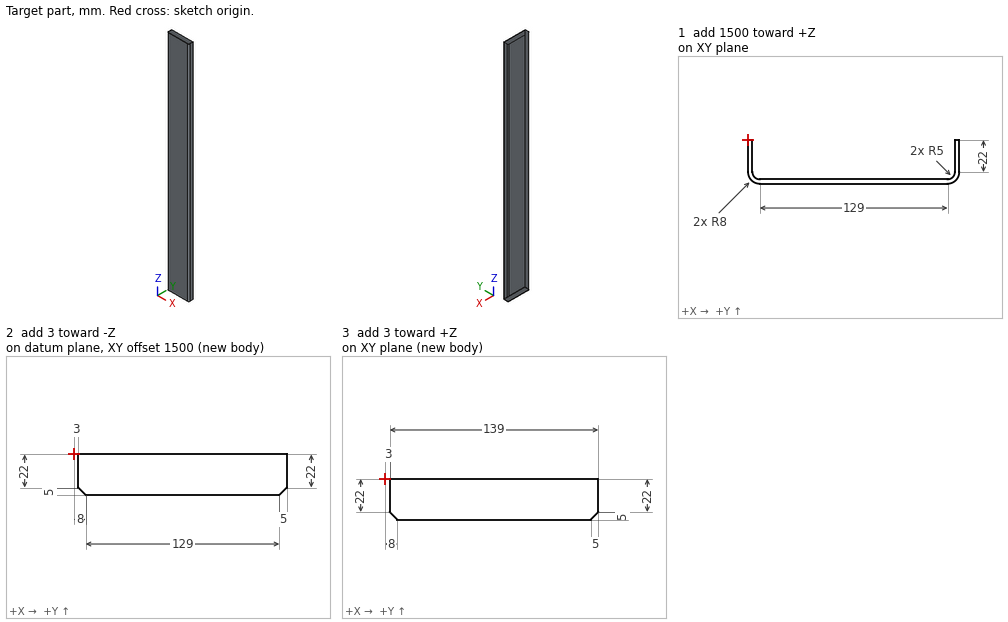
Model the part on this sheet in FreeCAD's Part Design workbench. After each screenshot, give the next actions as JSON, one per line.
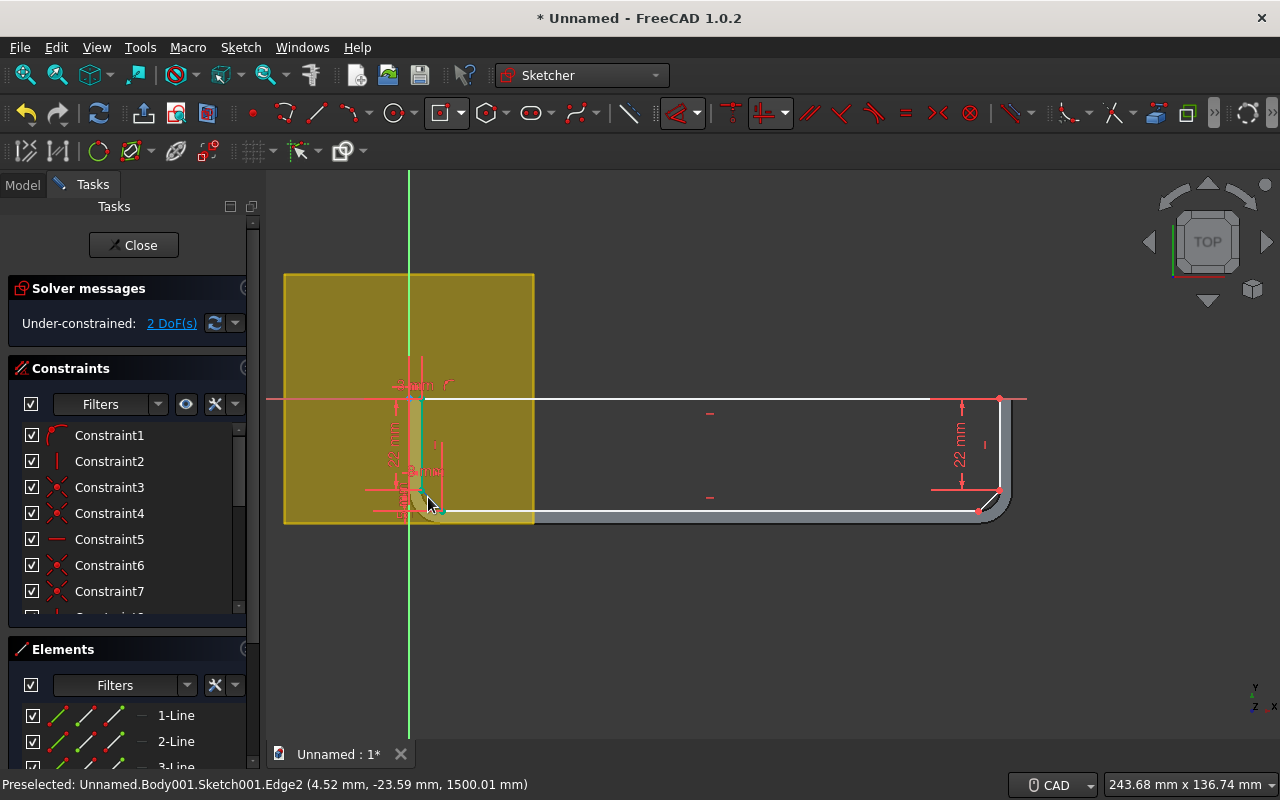
{"action": "scroll", "coordinate": [985, 505], "scroll_direction": "up", "scroll_amount": 4}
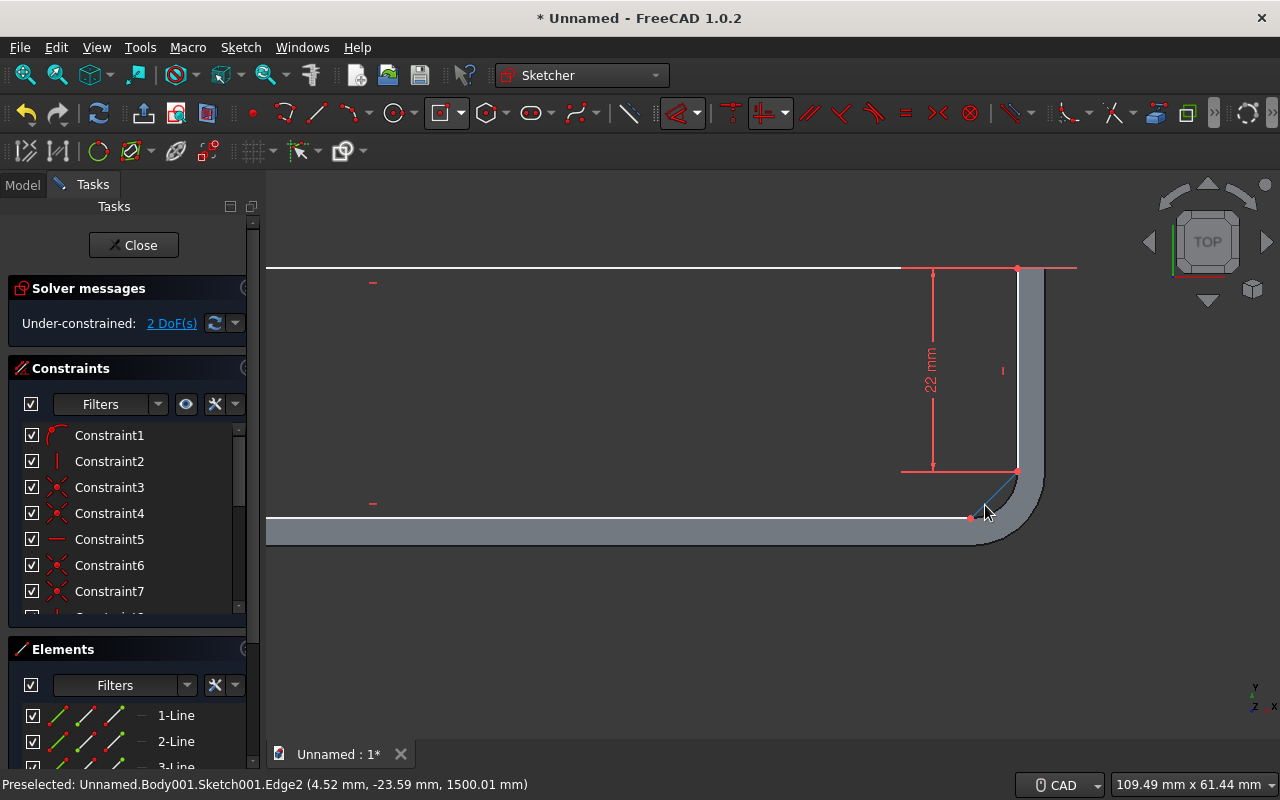
{"action": "left_click", "coordinate": [985, 504]}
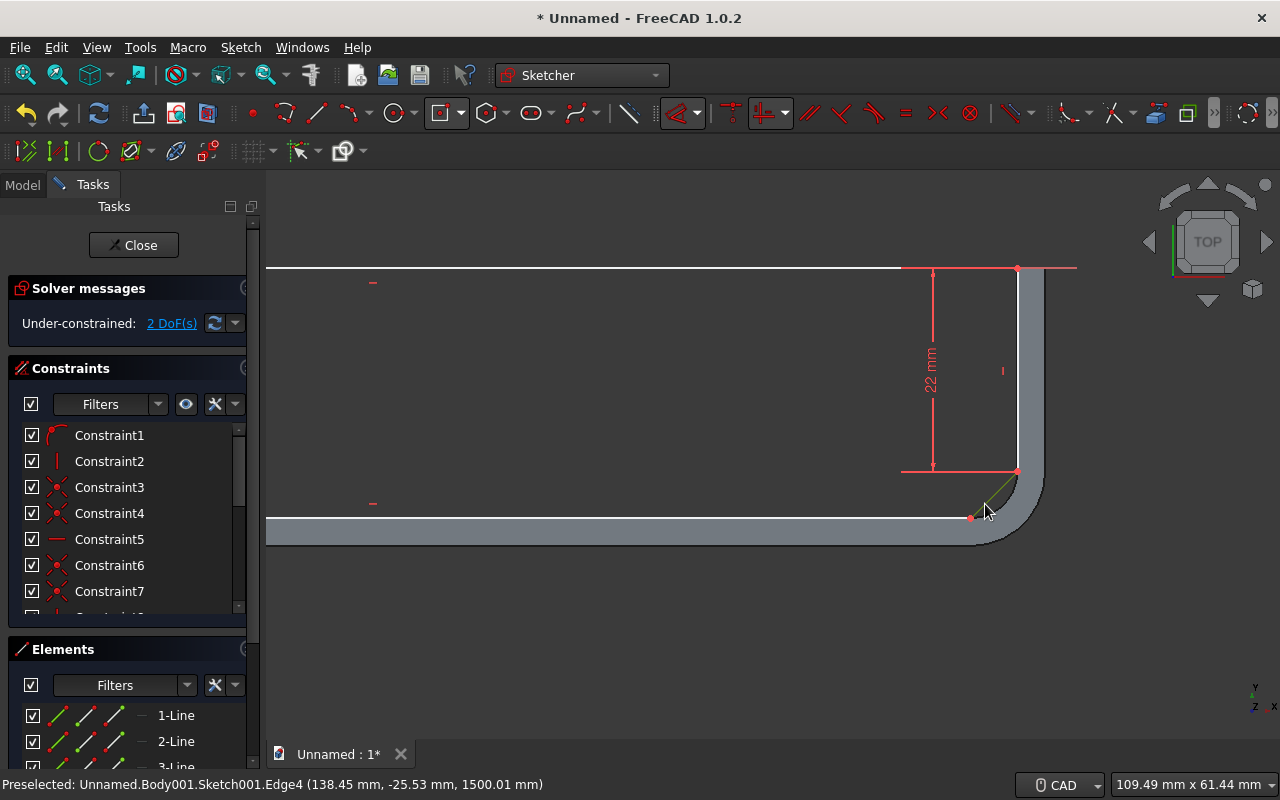
{"action": "key", "text": "l"}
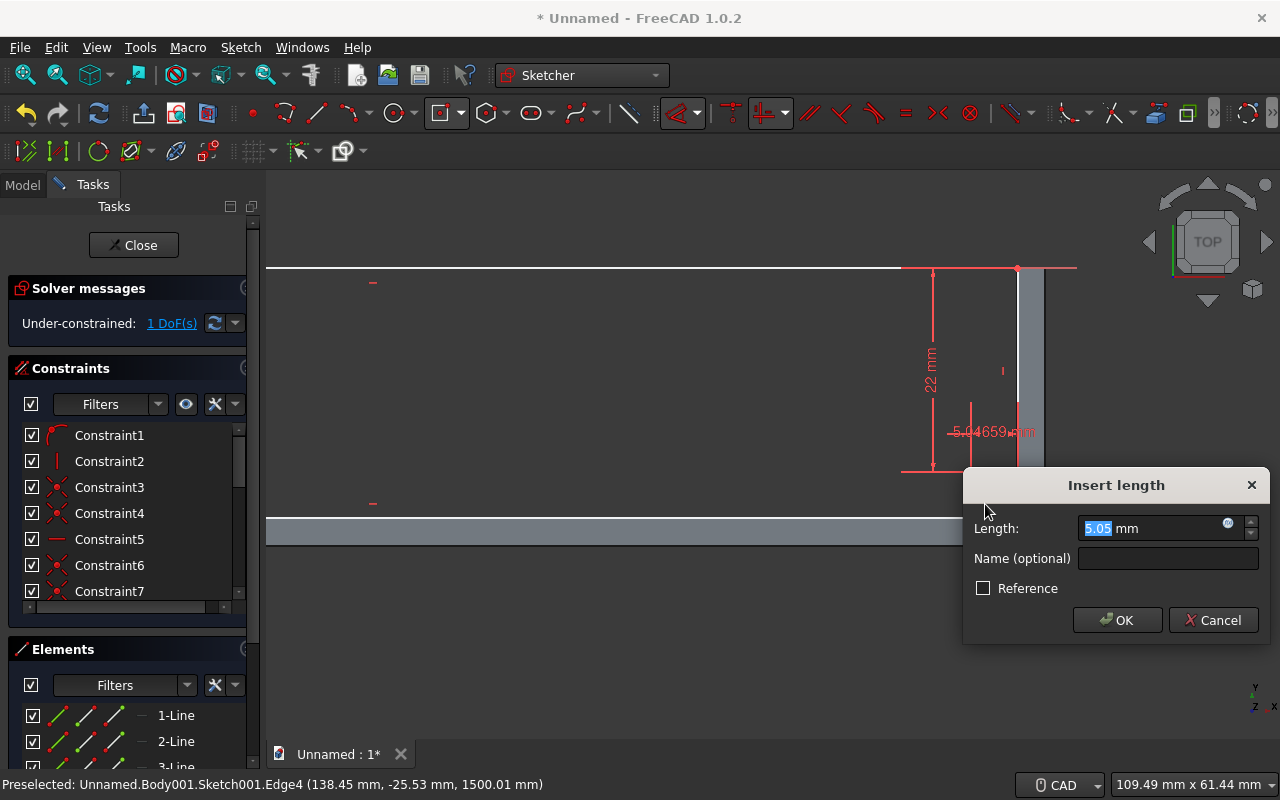
{"action": "type", "text": "5"}
{"action": "key", "text": "Return"}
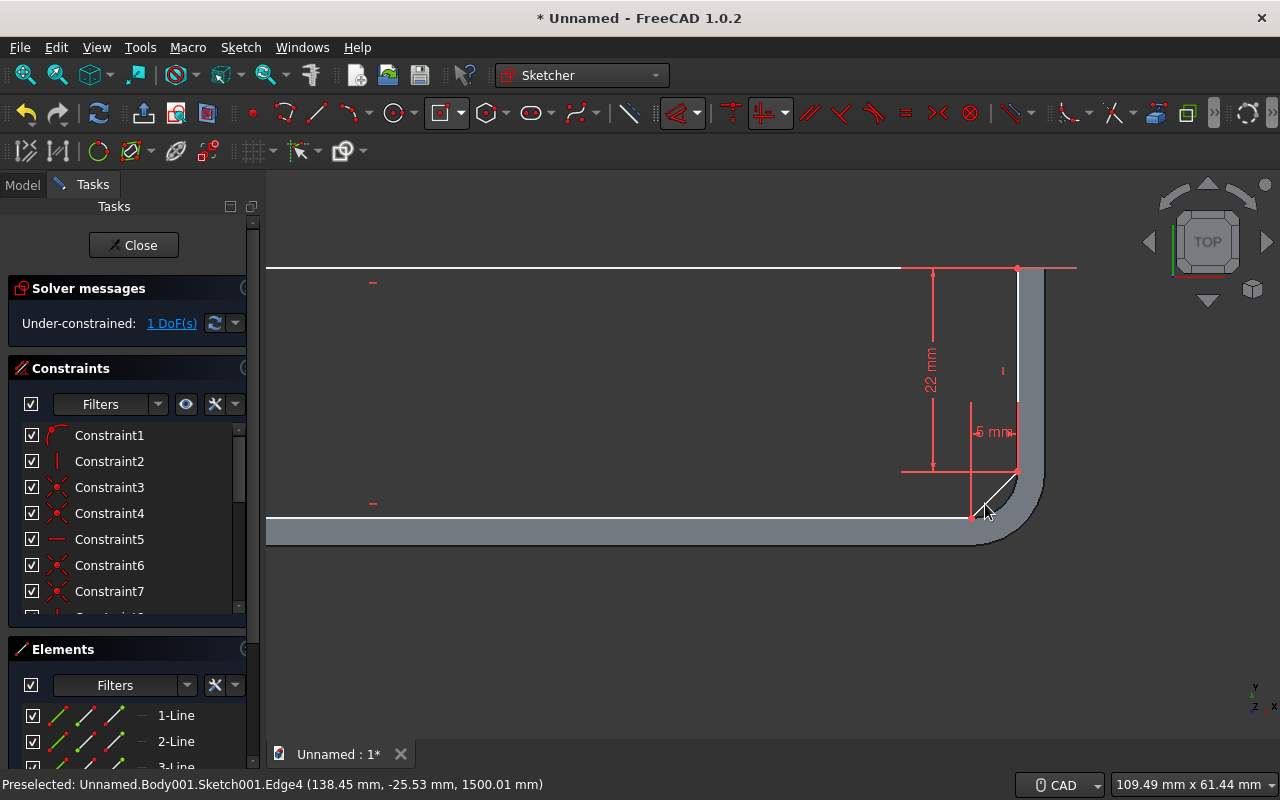
{"action": "left_click", "coordinate": [613, 518]}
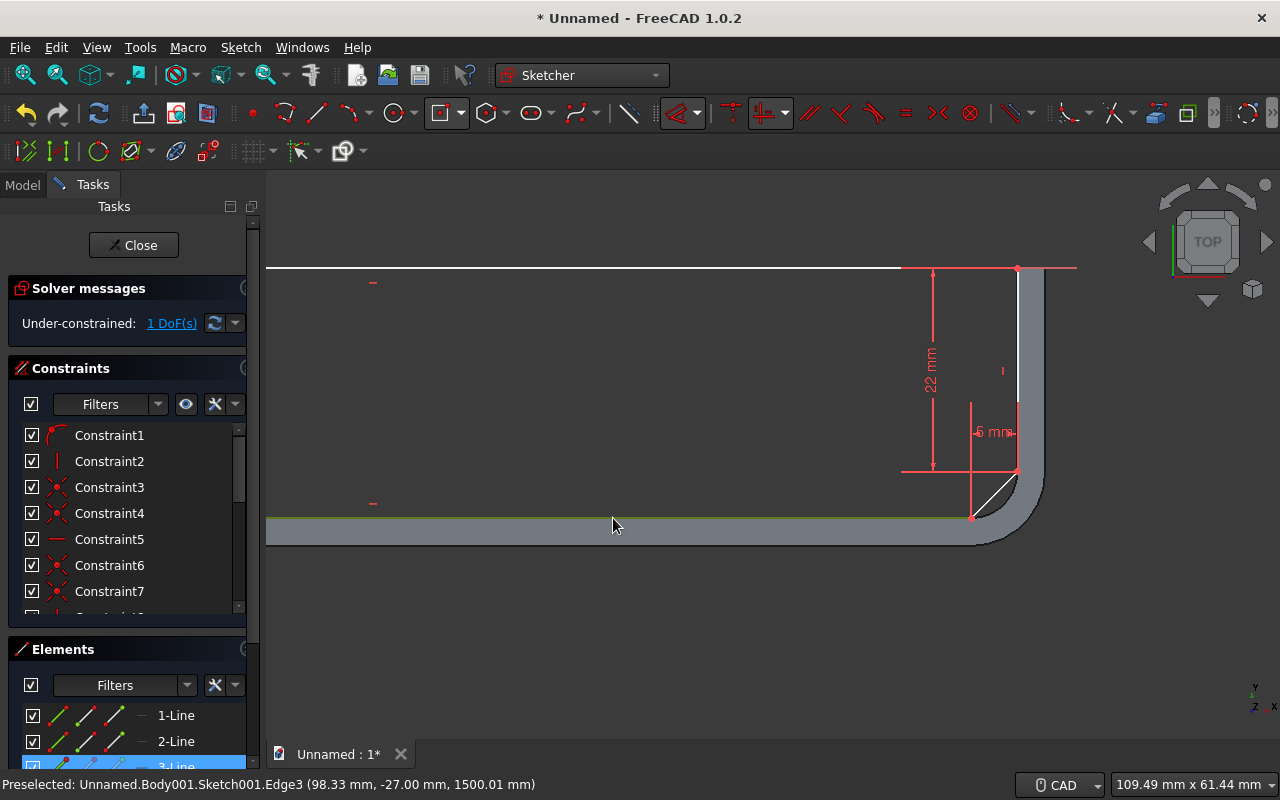
{"action": "key", "text": "l"}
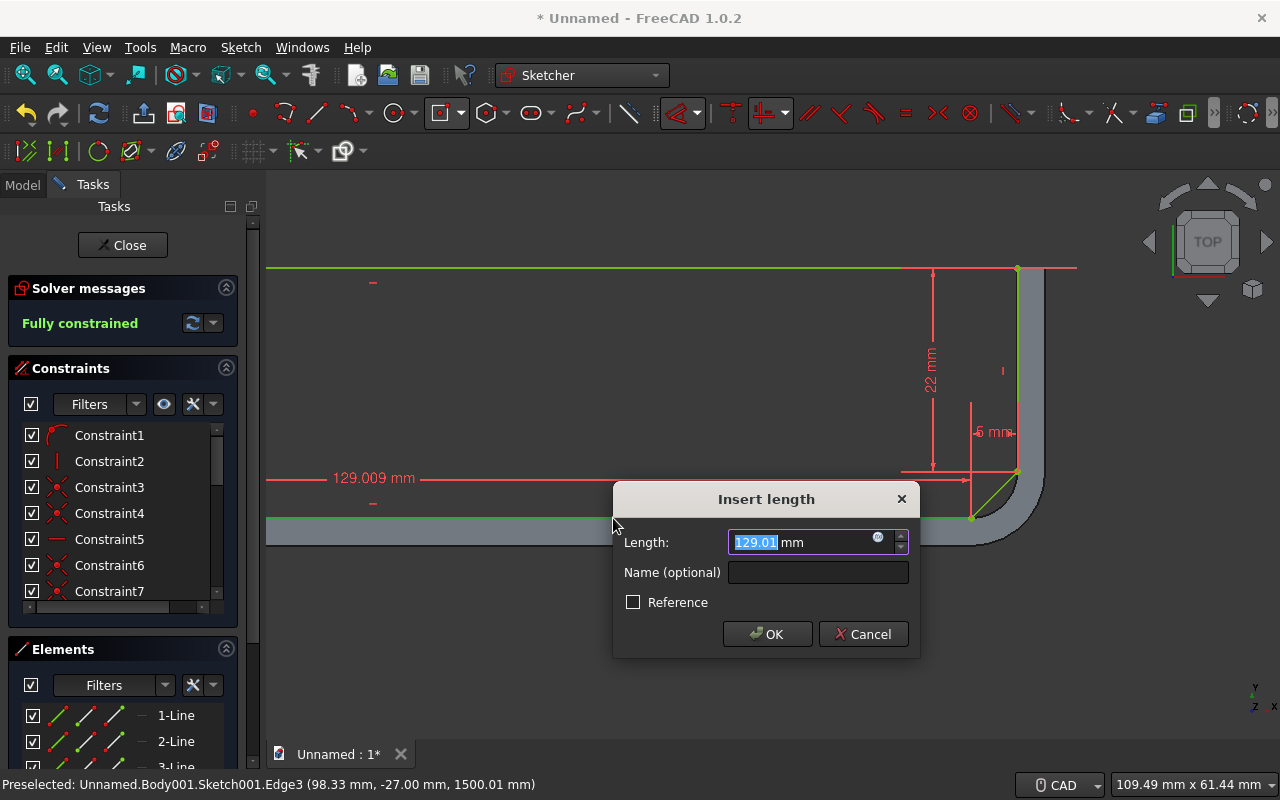
{"action": "type", "text": "129"}
{"action": "key", "text": "Return"}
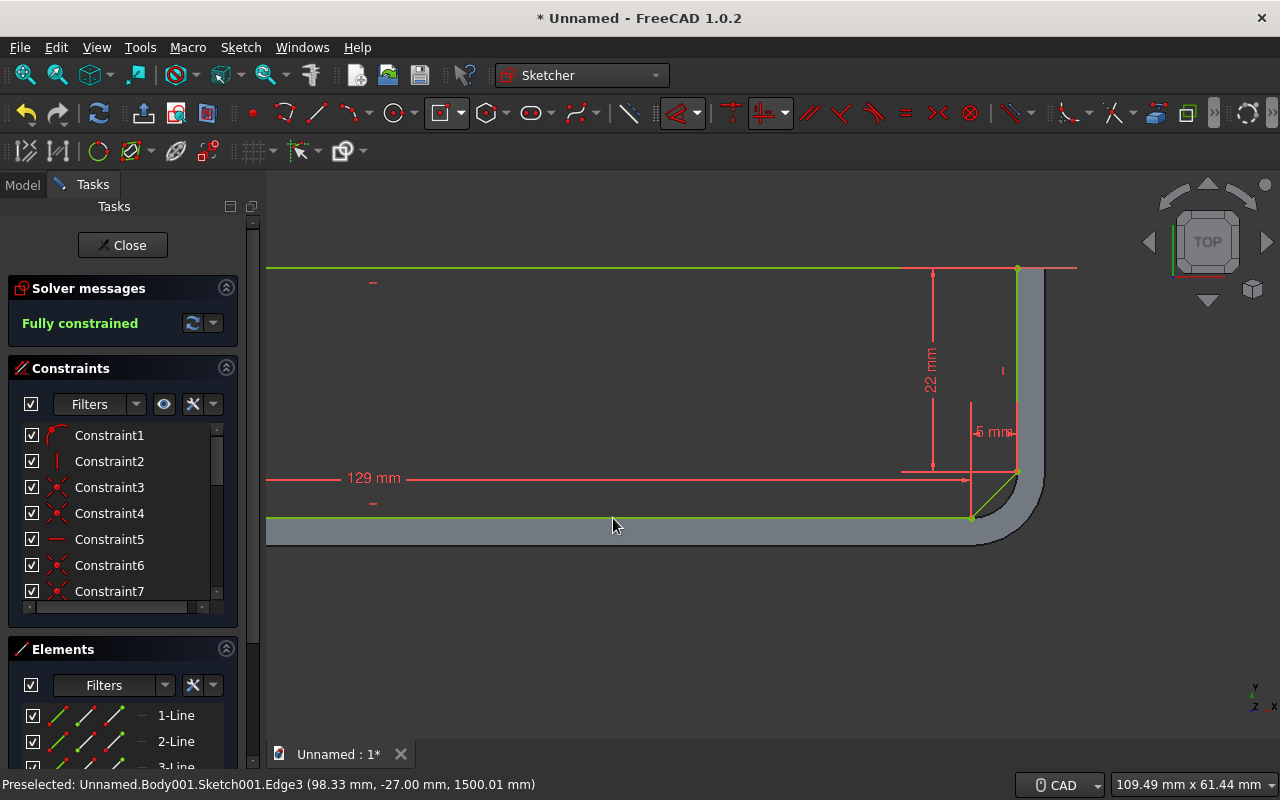
{"action": "left_click", "coordinate": [123, 245]}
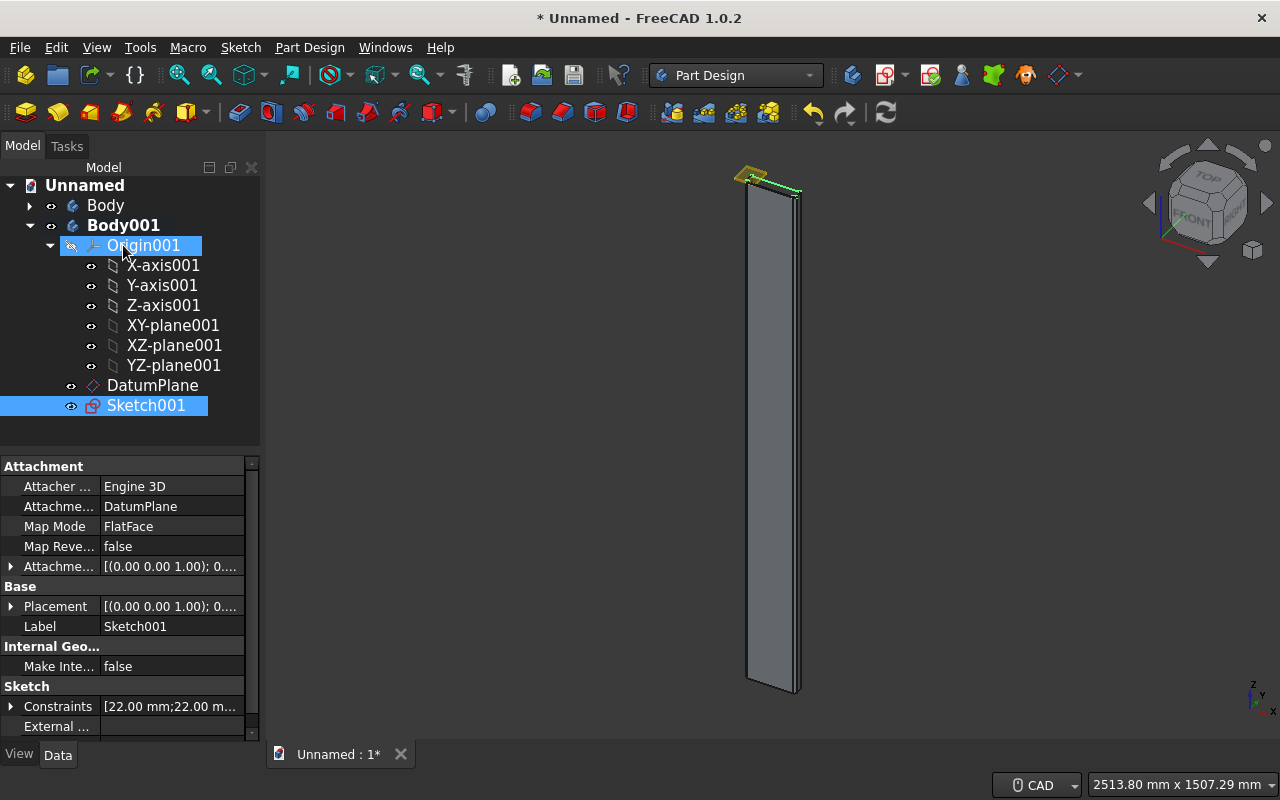
{"action": "left_click", "coordinate": [26, 112]}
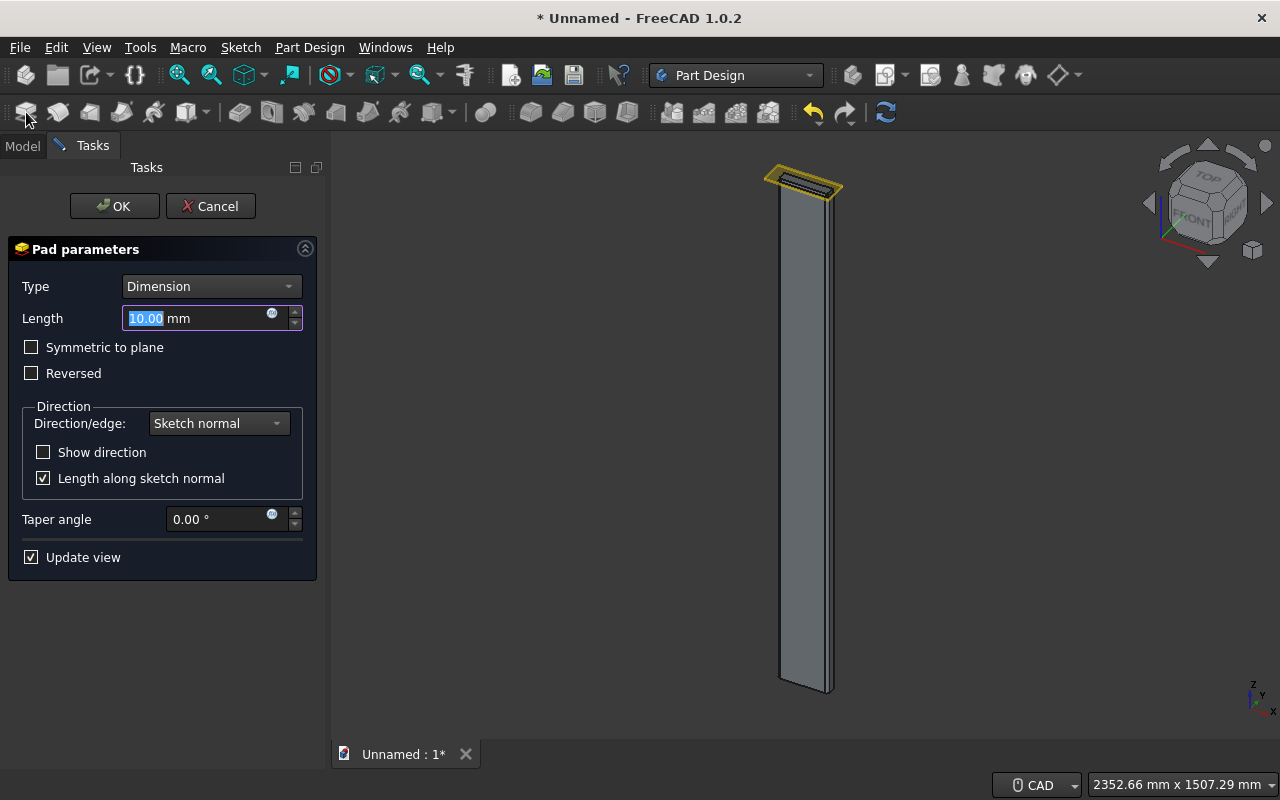
{"action": "type", "text": "3"}
{"action": "key", "text": "Tab"}